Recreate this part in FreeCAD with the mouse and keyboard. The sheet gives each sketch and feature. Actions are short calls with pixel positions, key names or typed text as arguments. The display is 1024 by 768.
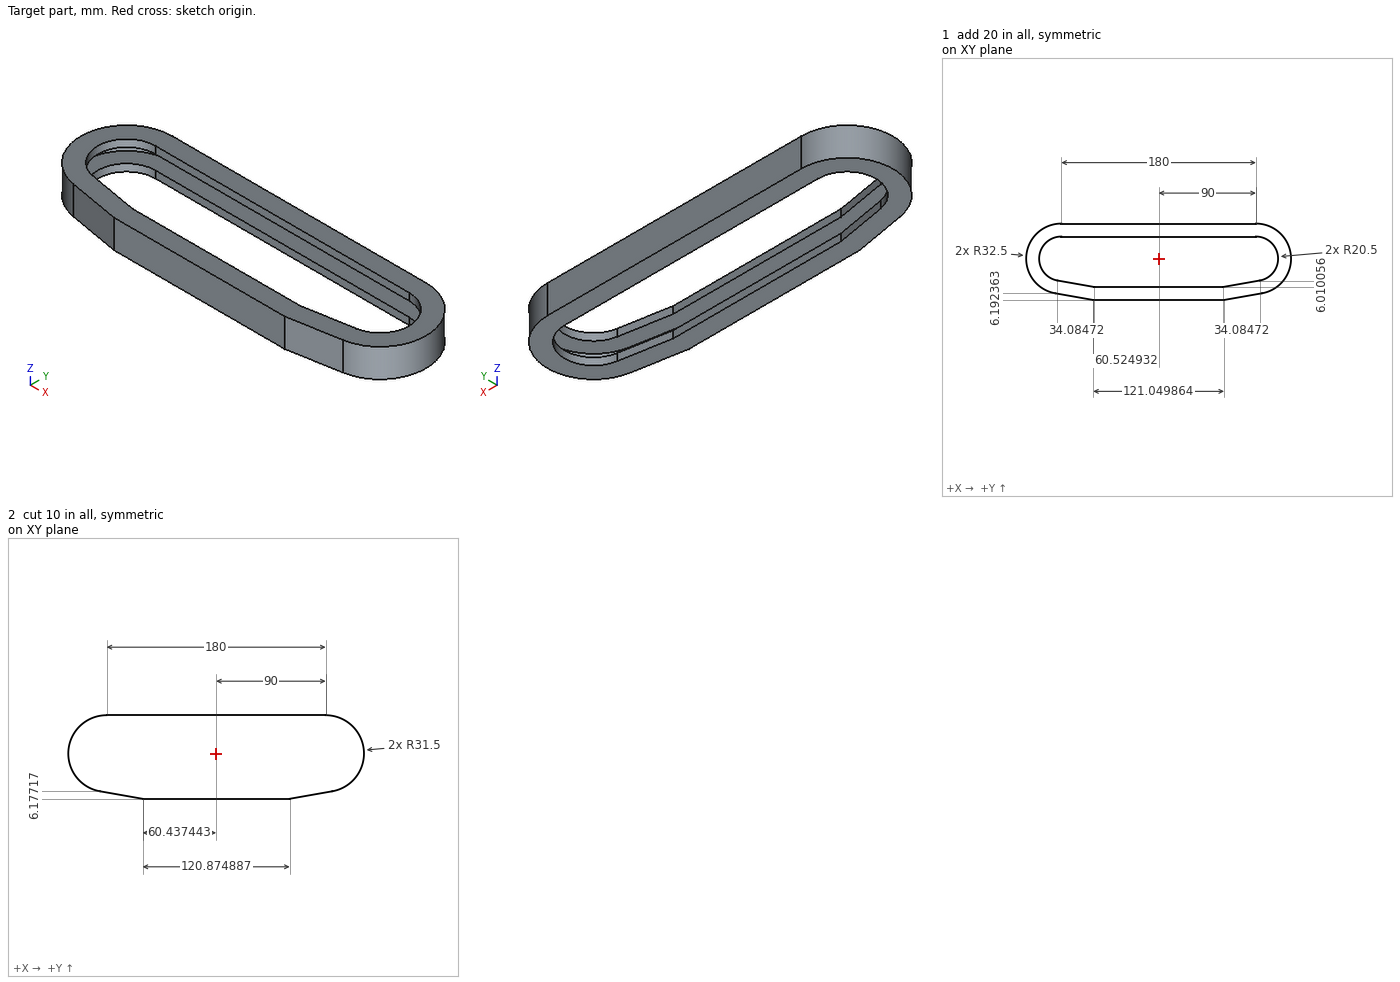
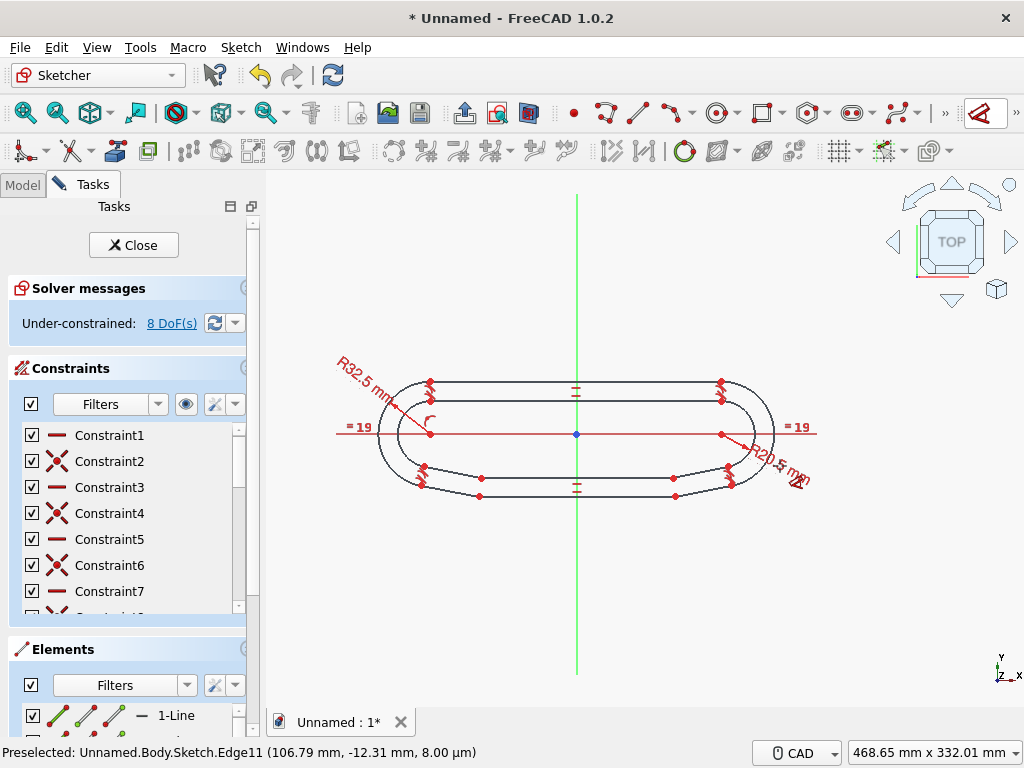
click(634, 382)
click(509, 348)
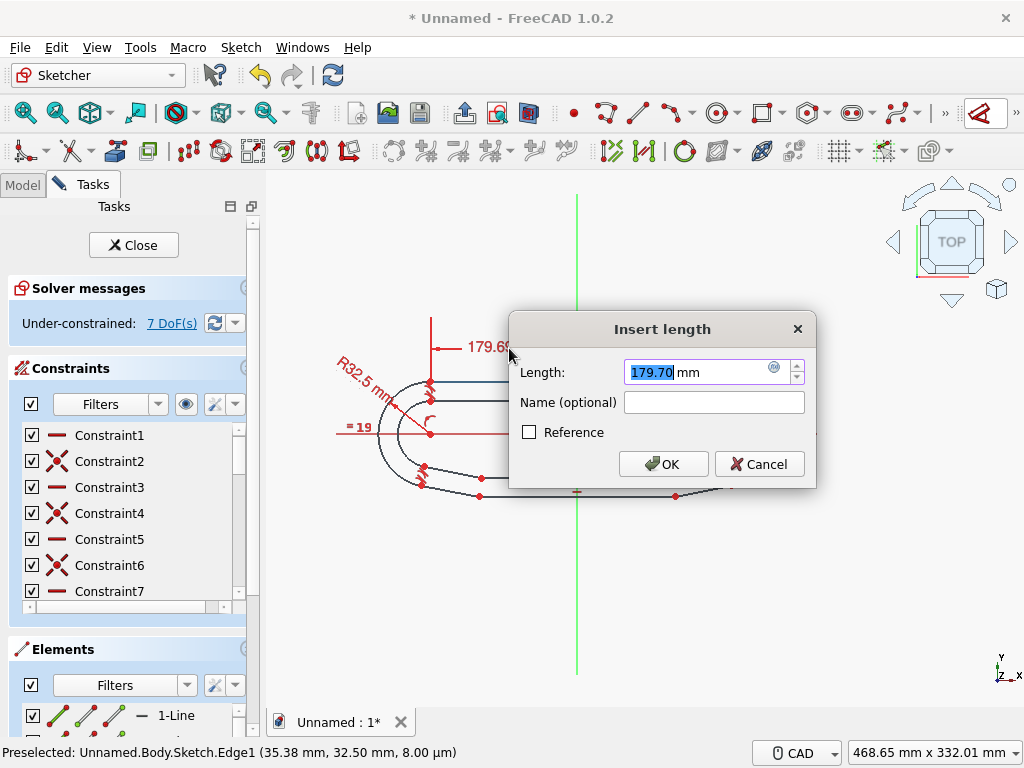
text(180)
key(Return)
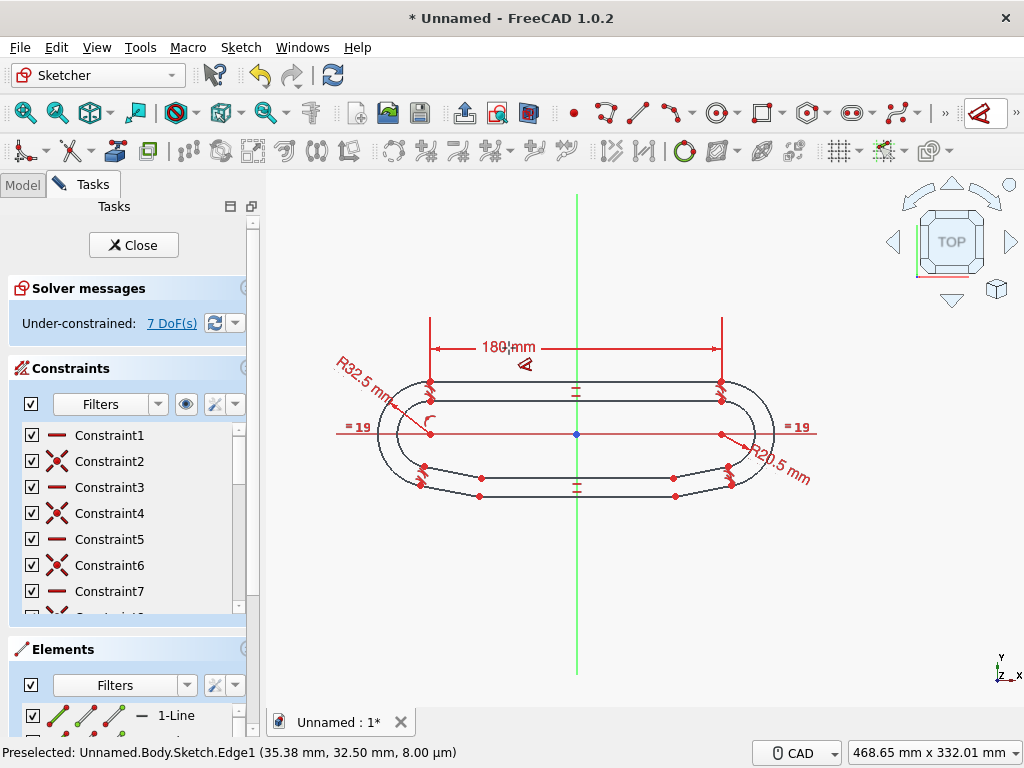
click(722, 382)
click(649, 348)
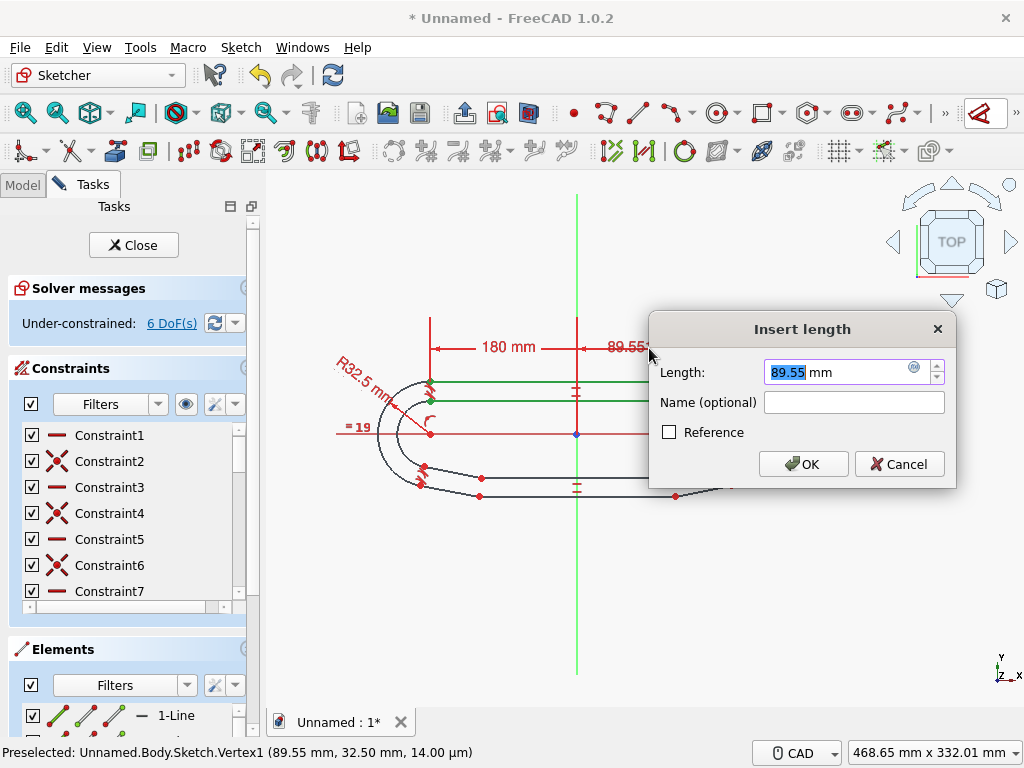
text(90)
key(Return)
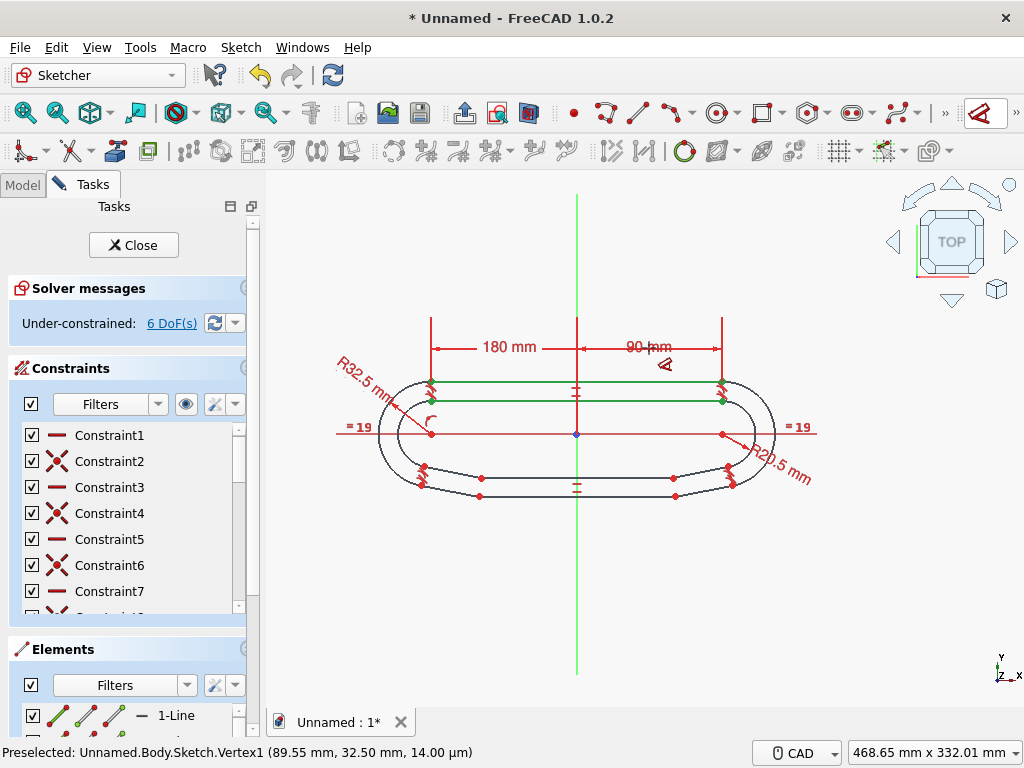
scroll(439, 489, up, 7)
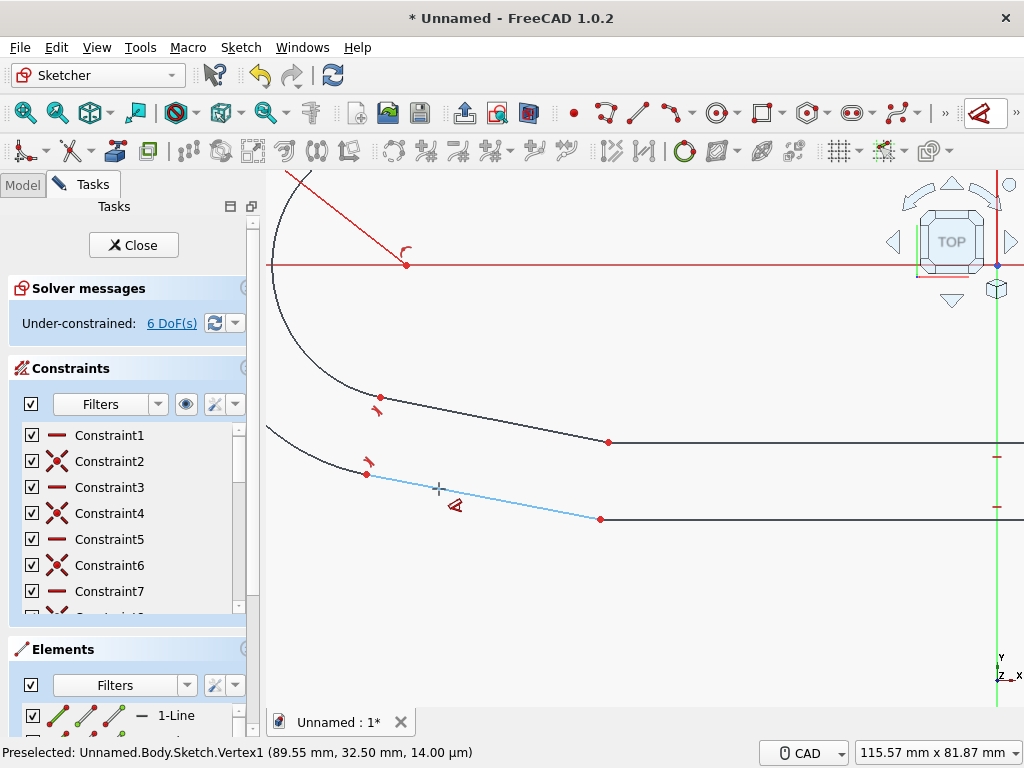
click(437, 488)
click(333, 497)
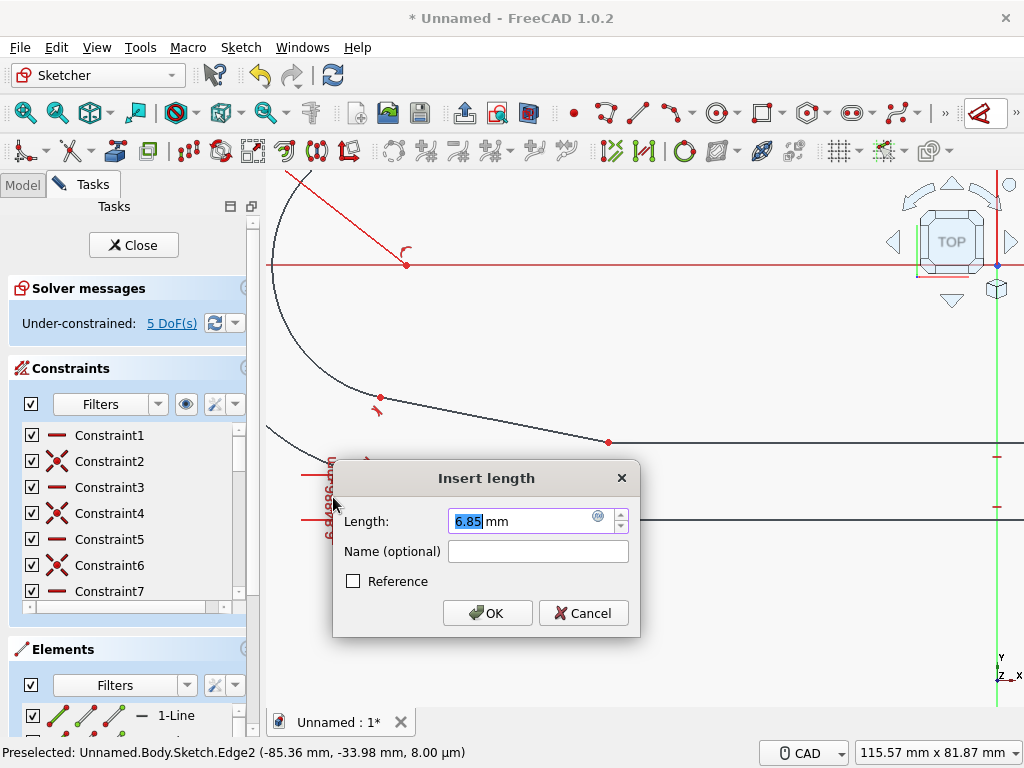
text(6.192363)
key(Return)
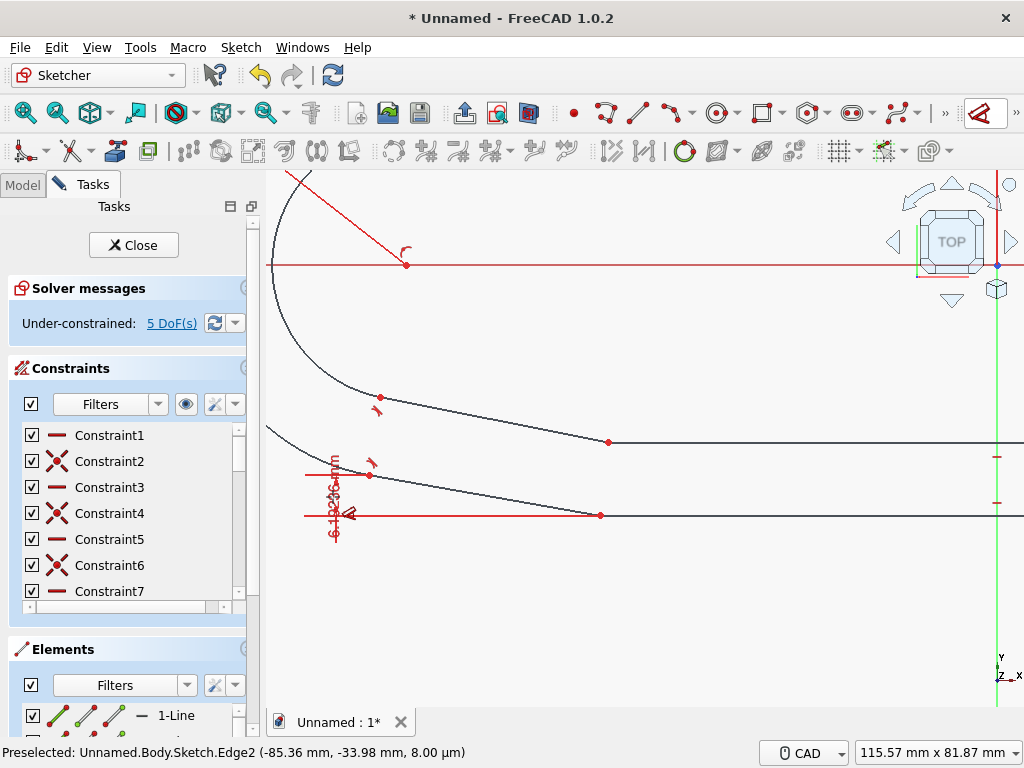
scroll(439, 489, down, 7)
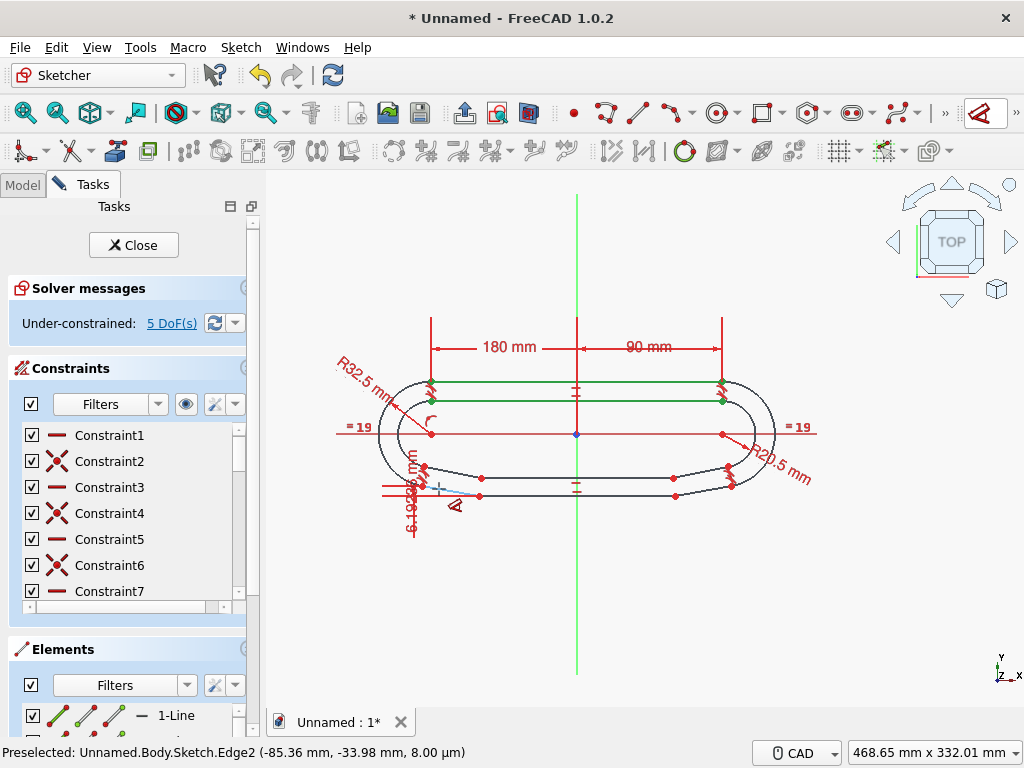
click(712, 470)
click(701, 512)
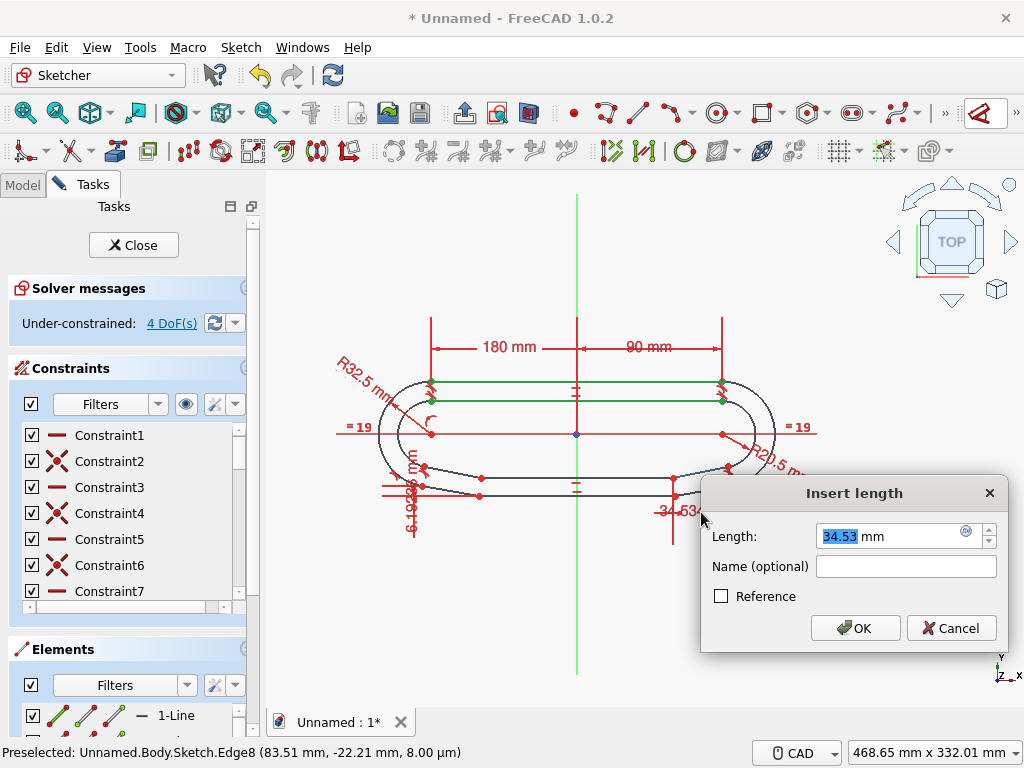
text(34.08472)
key(Return)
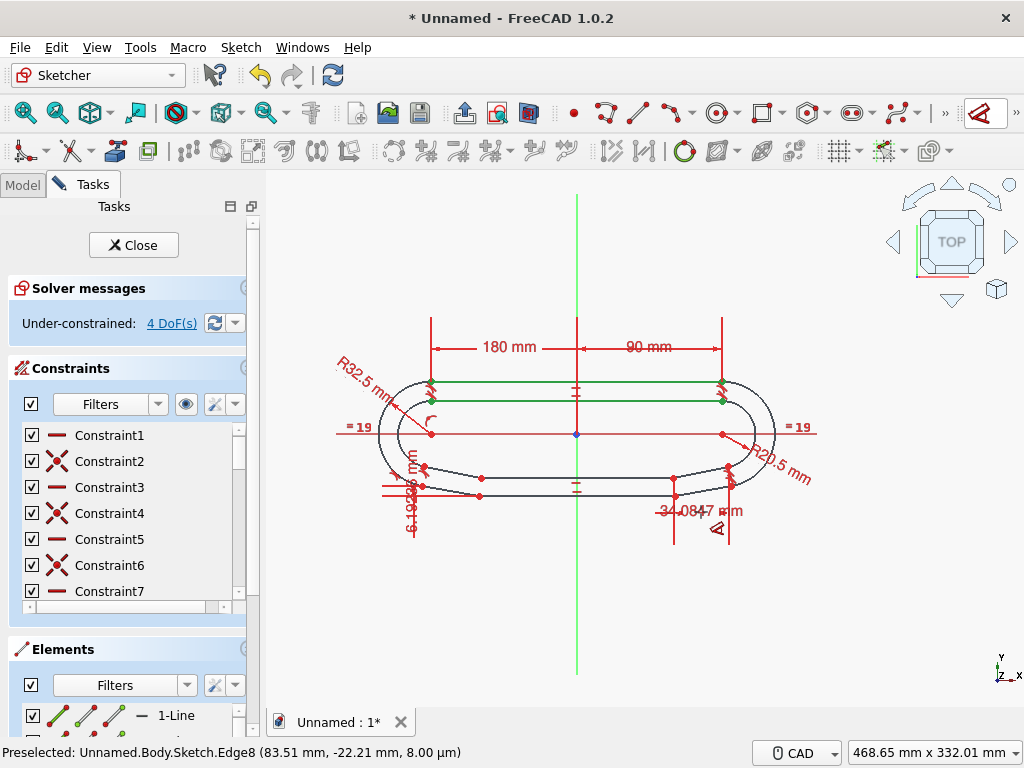
scroll(712, 470, up, 8)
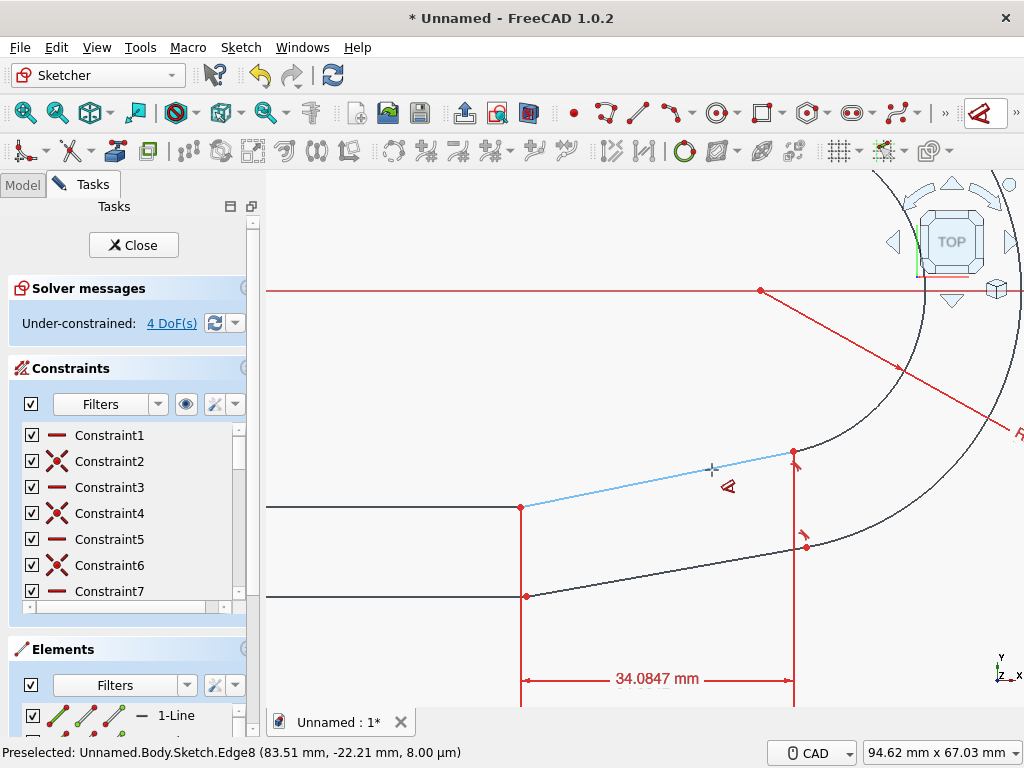
click(712, 469)
click(828, 480)